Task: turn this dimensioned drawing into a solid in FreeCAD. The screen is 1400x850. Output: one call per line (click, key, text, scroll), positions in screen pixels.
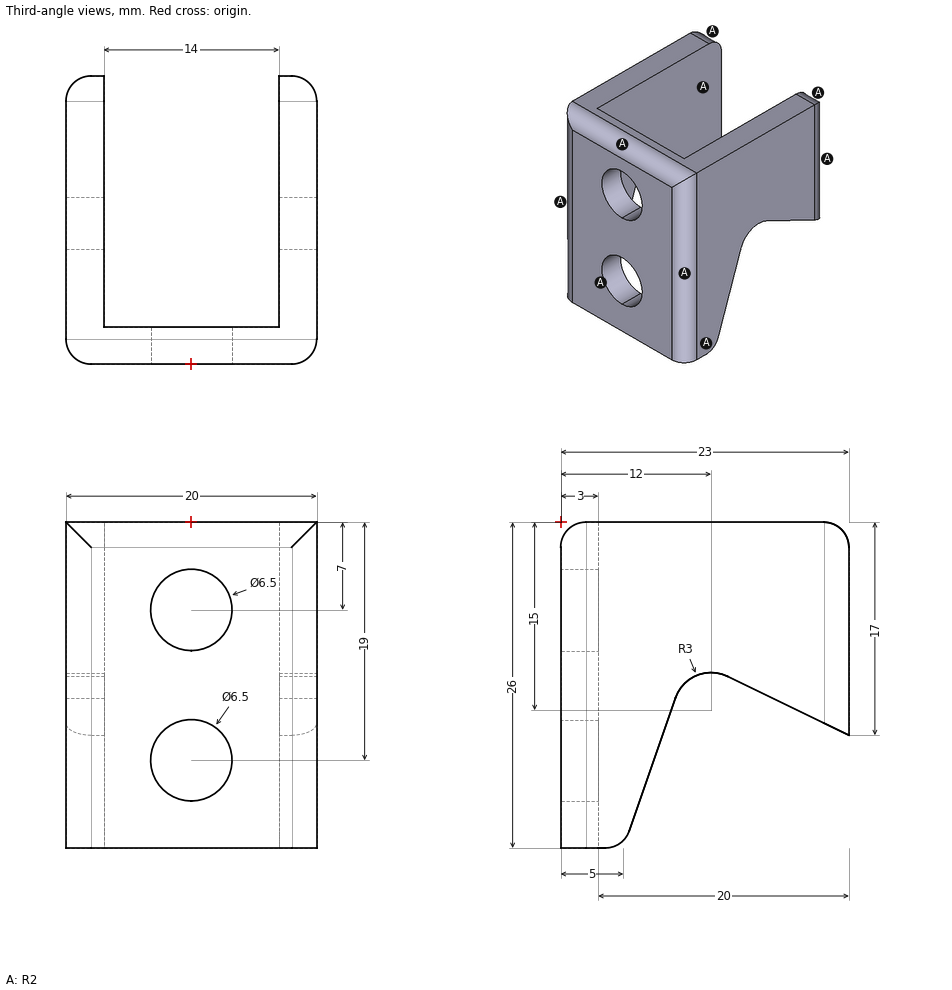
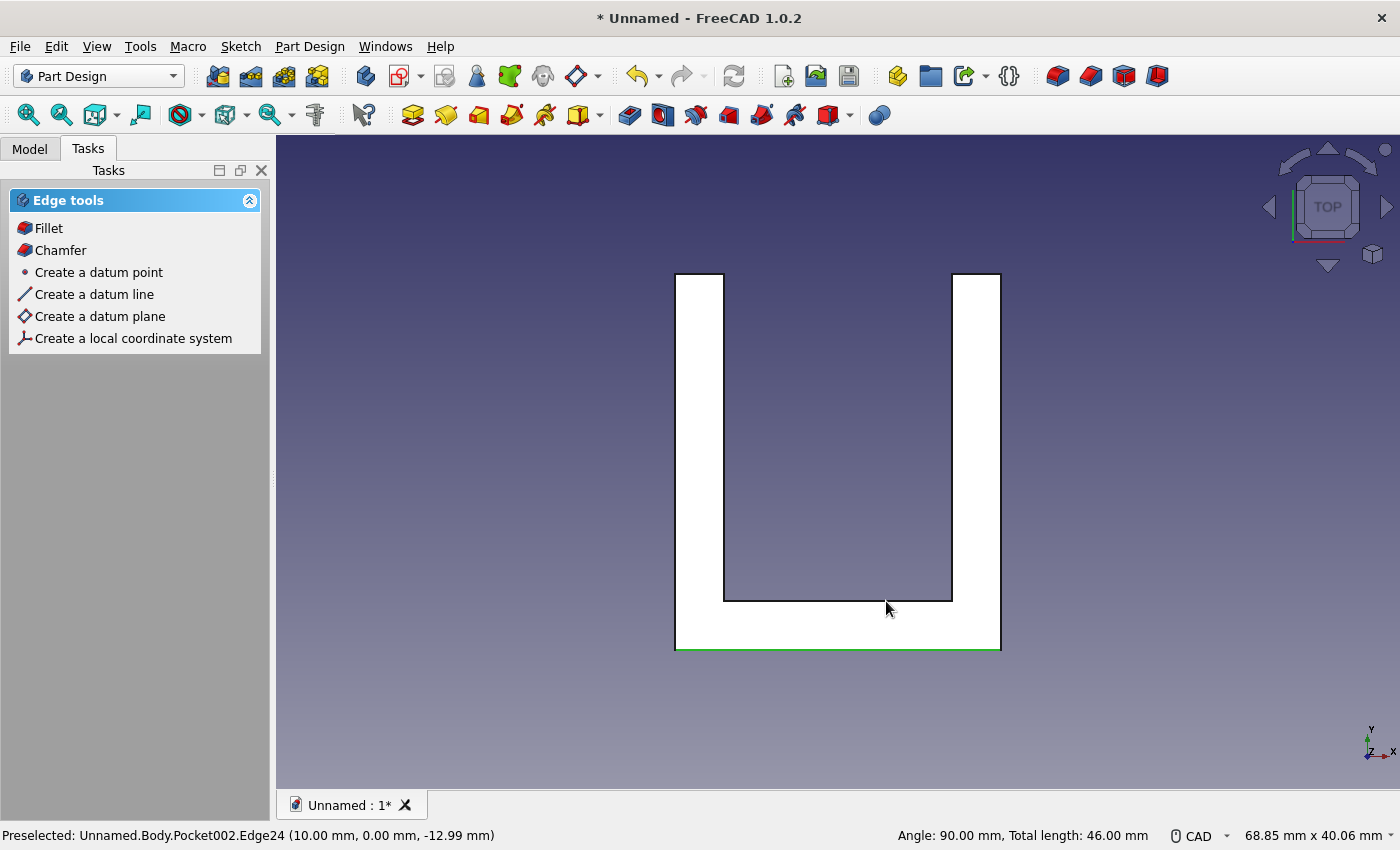
key(1)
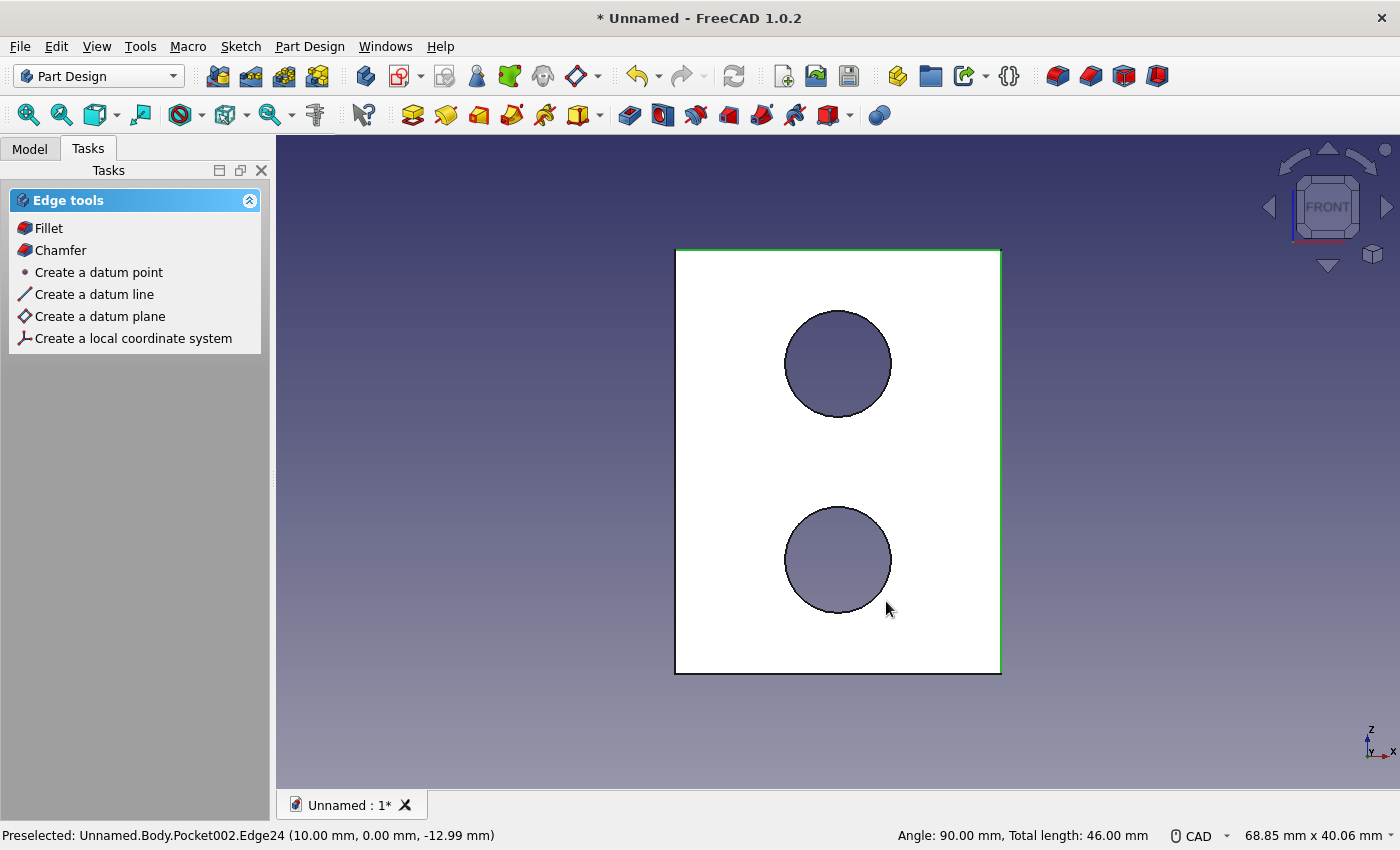
key(3)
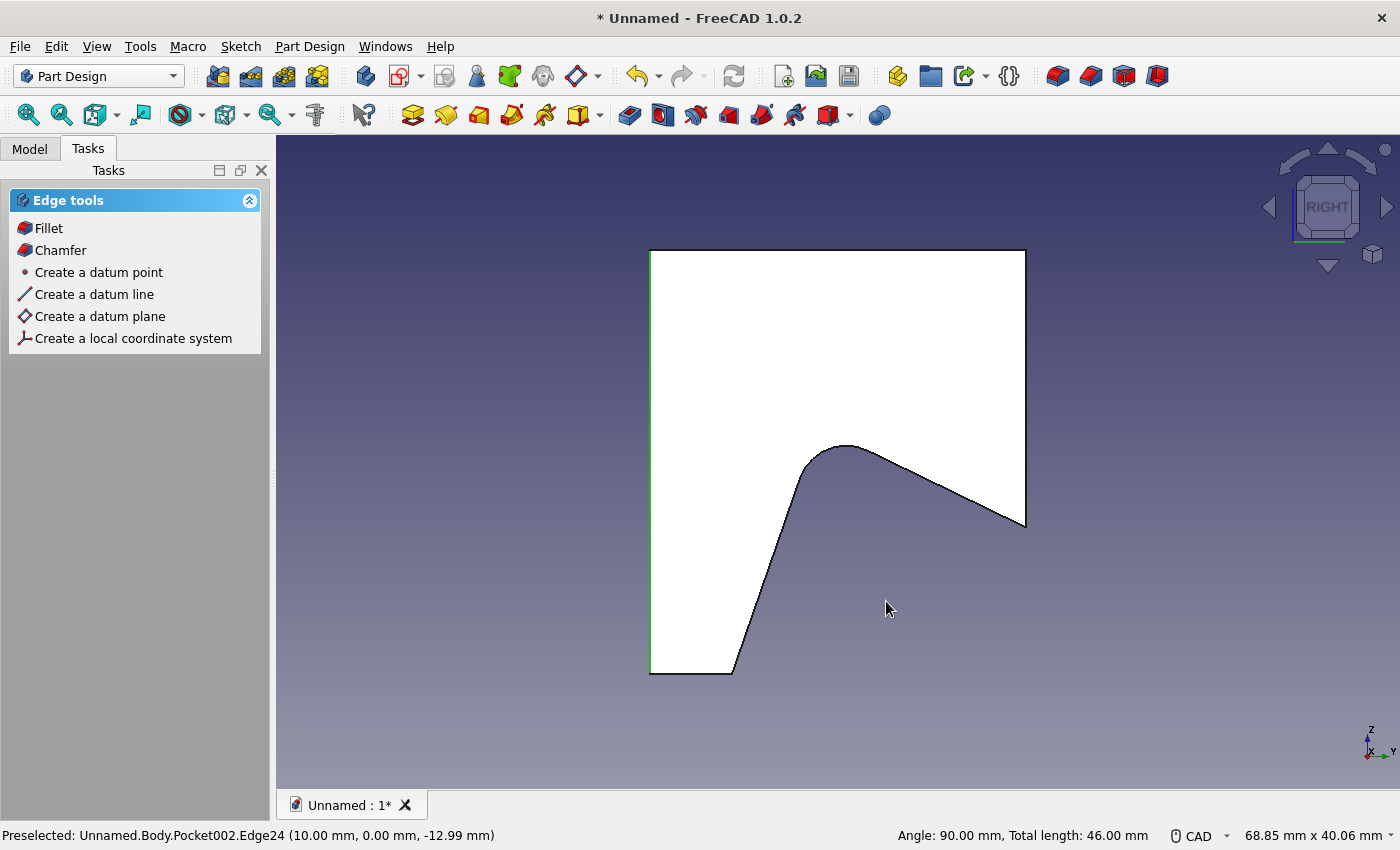
click(1026, 388, ctrl)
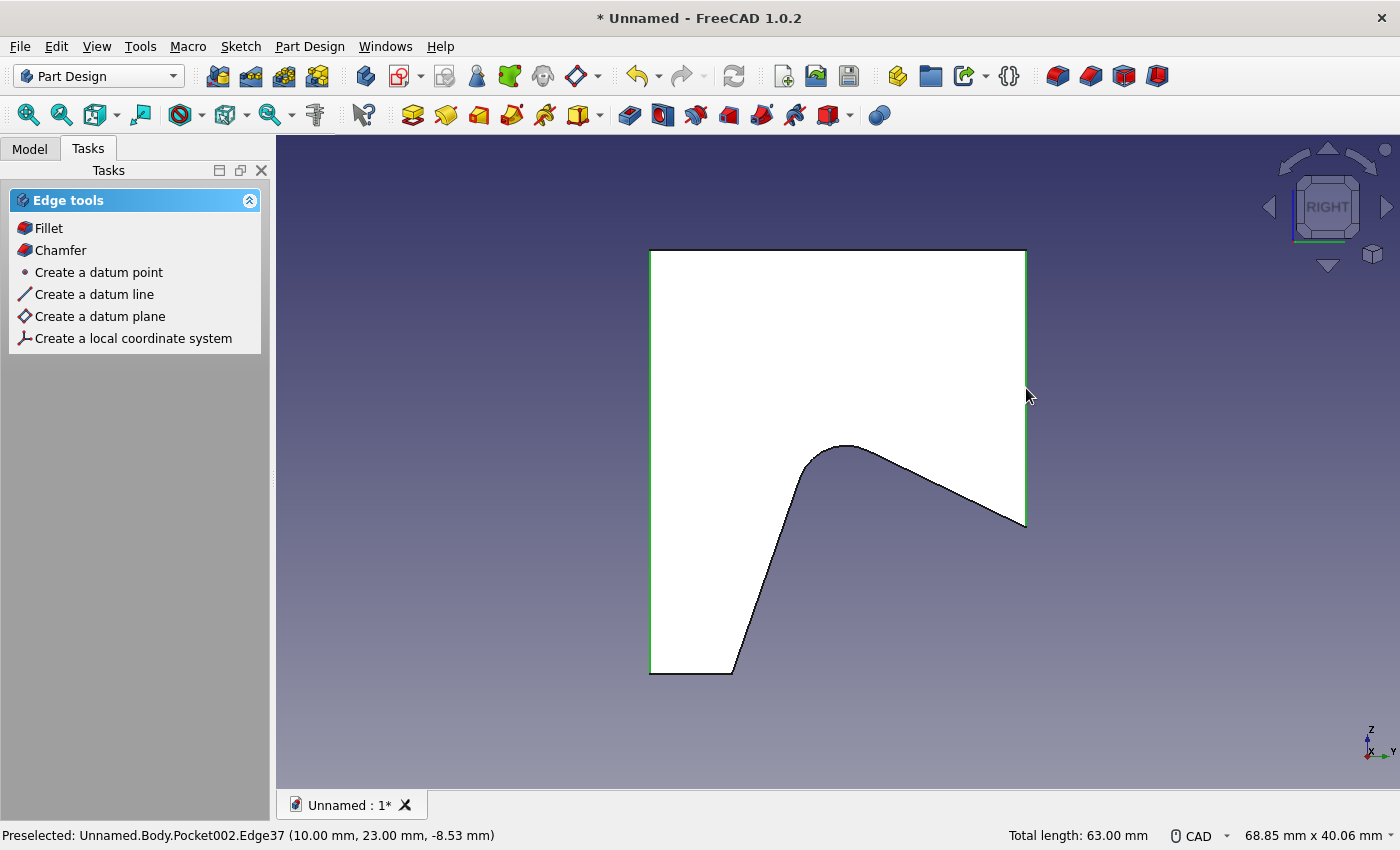
key(5)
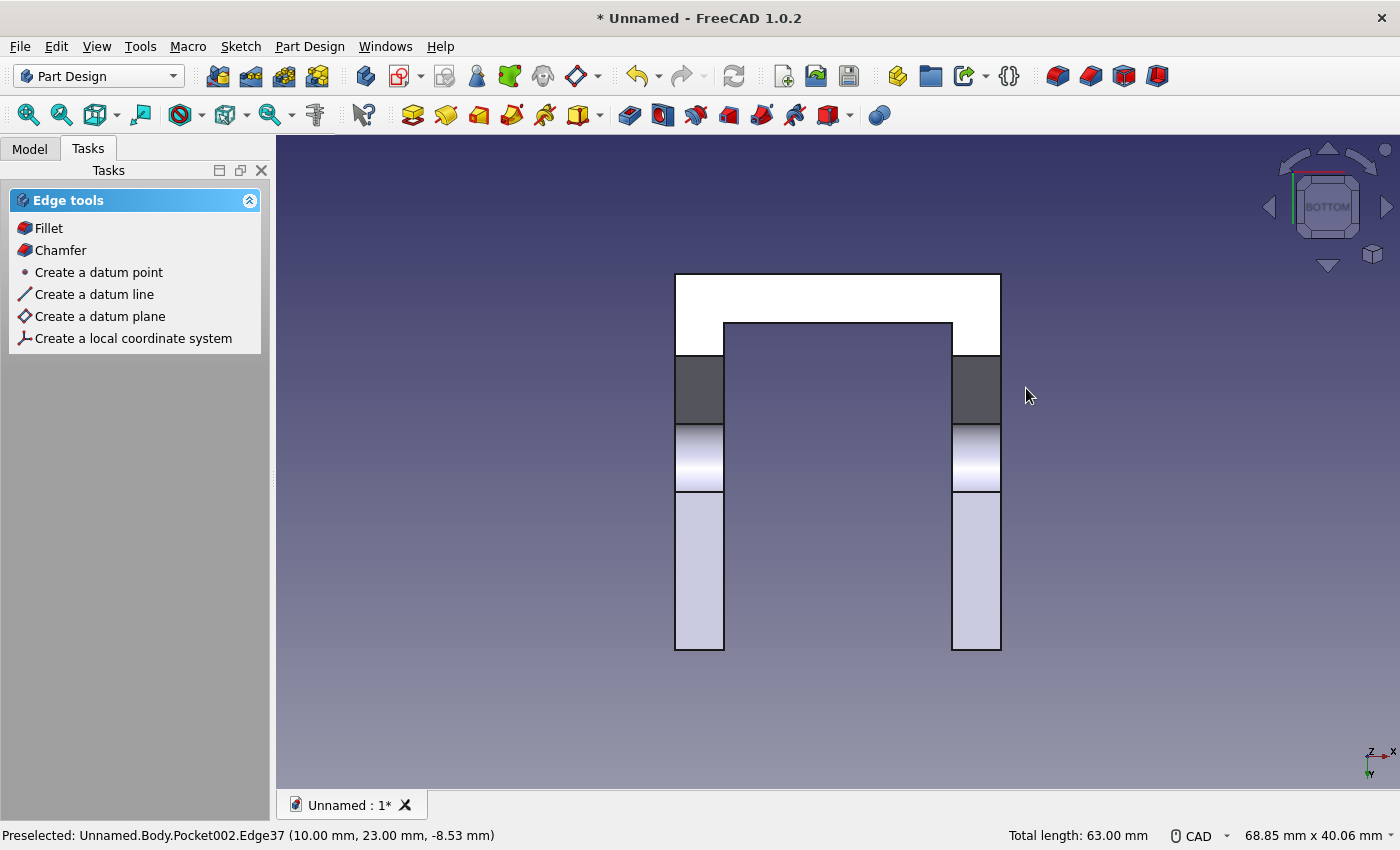
click(977, 355, ctrl)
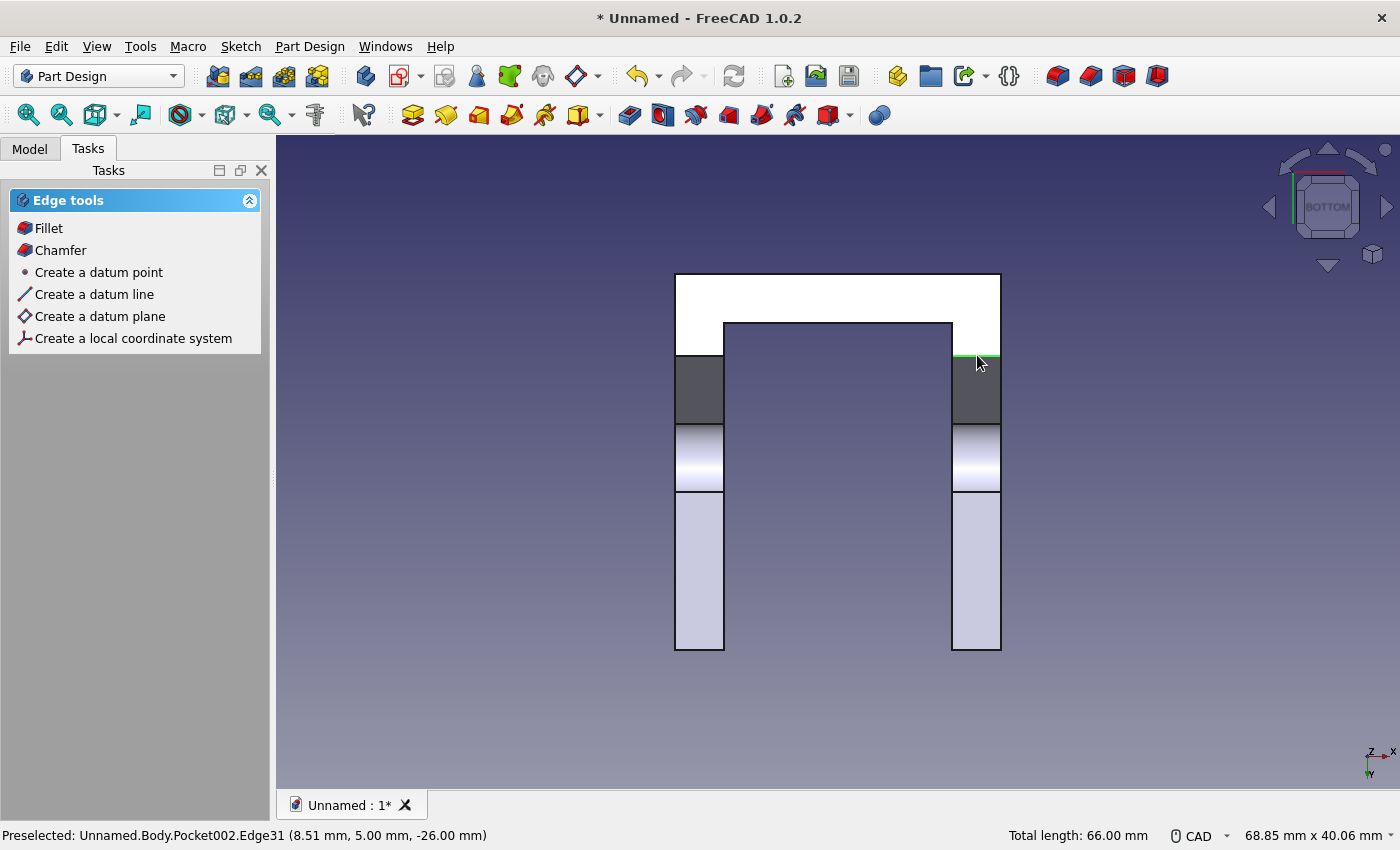
click(699, 355, ctrl)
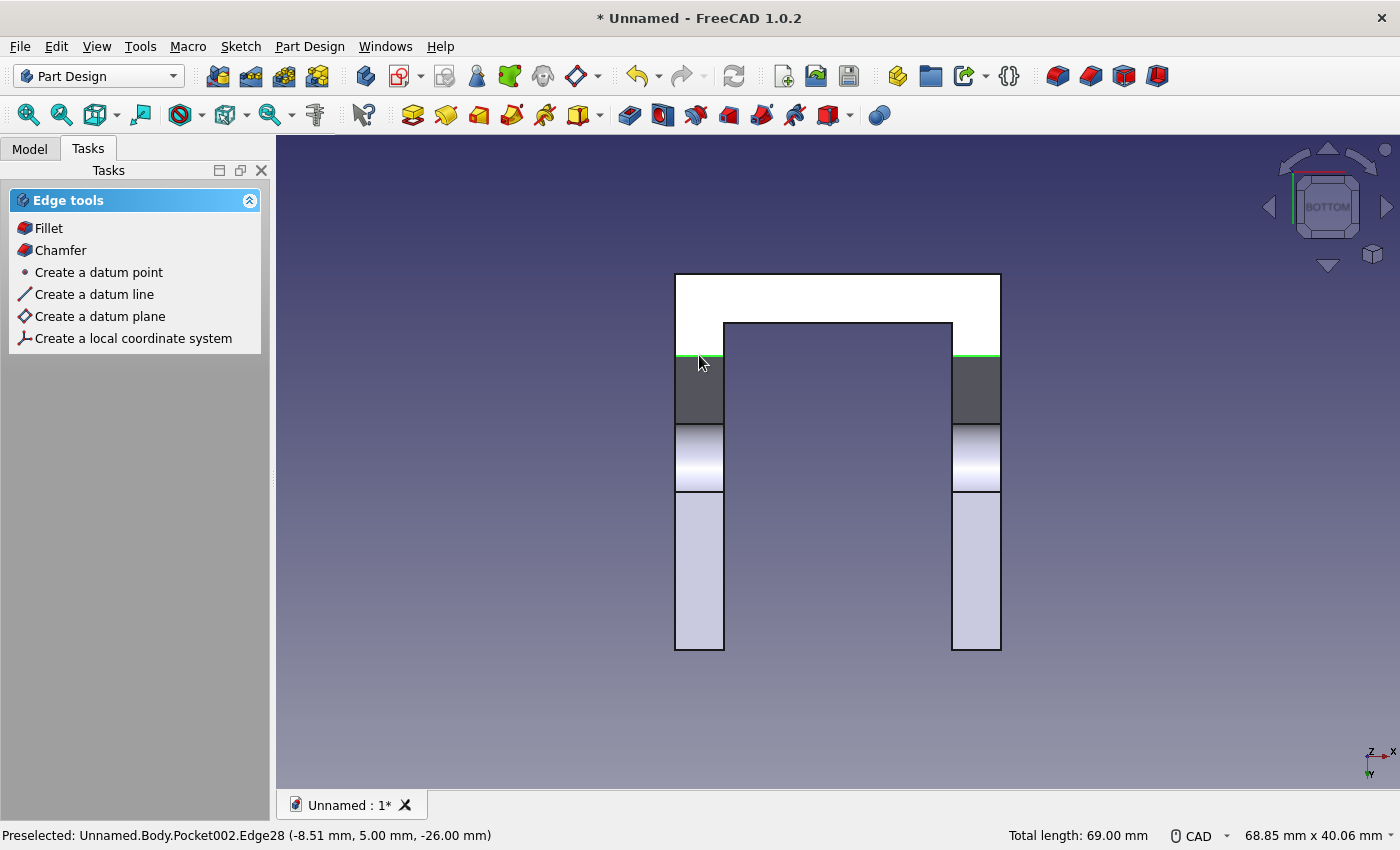
key(4)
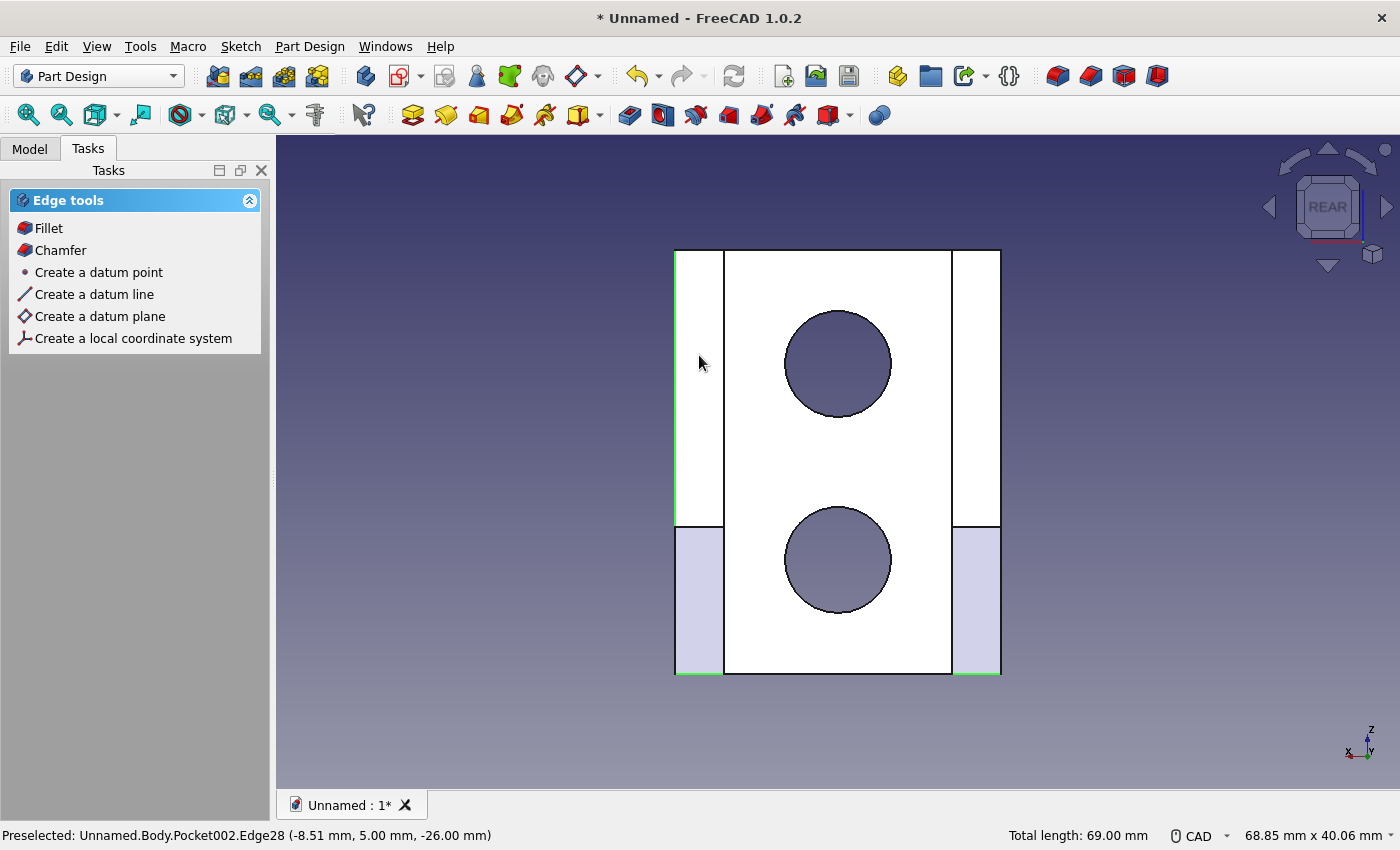
click(1001, 388, ctrl)